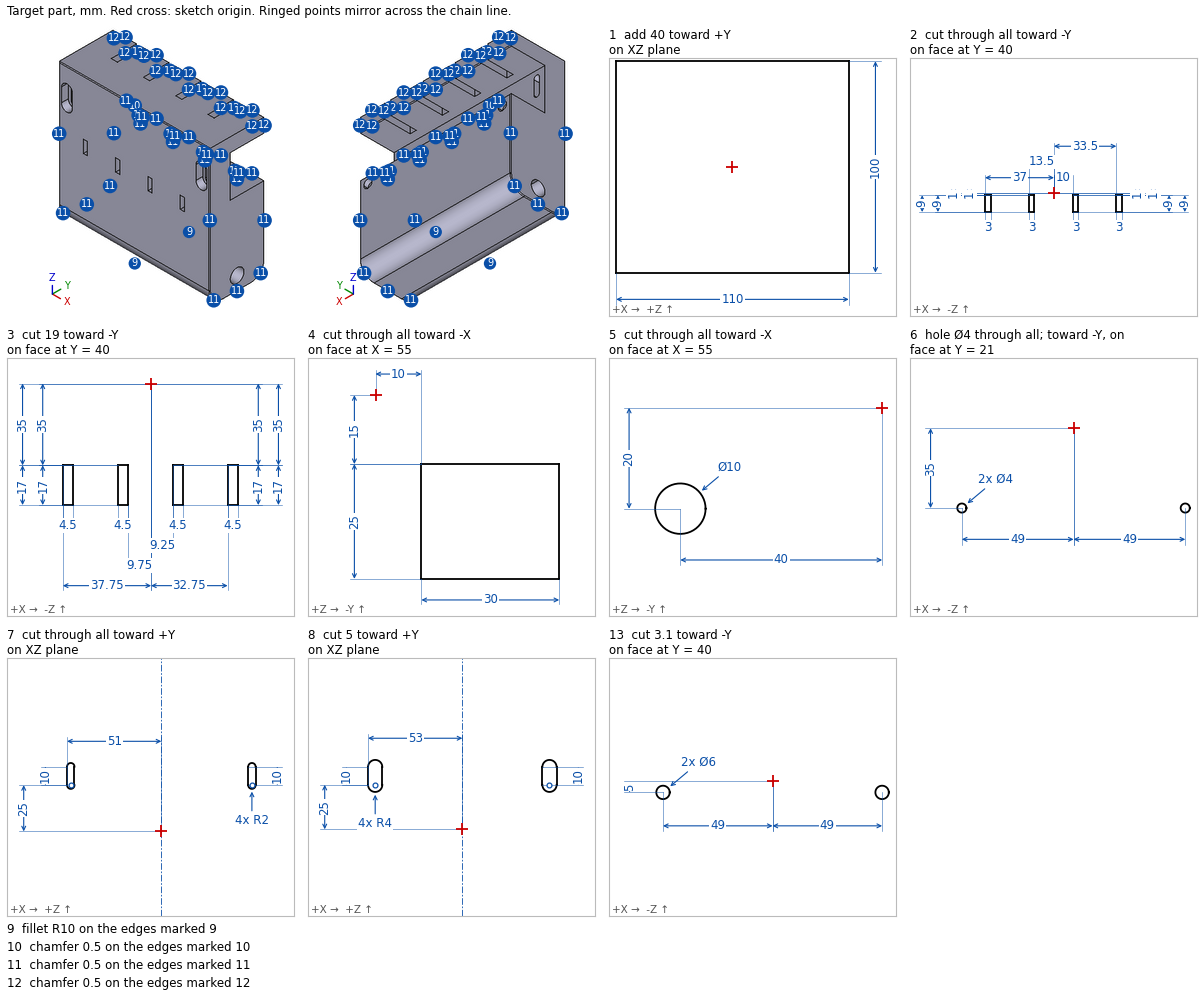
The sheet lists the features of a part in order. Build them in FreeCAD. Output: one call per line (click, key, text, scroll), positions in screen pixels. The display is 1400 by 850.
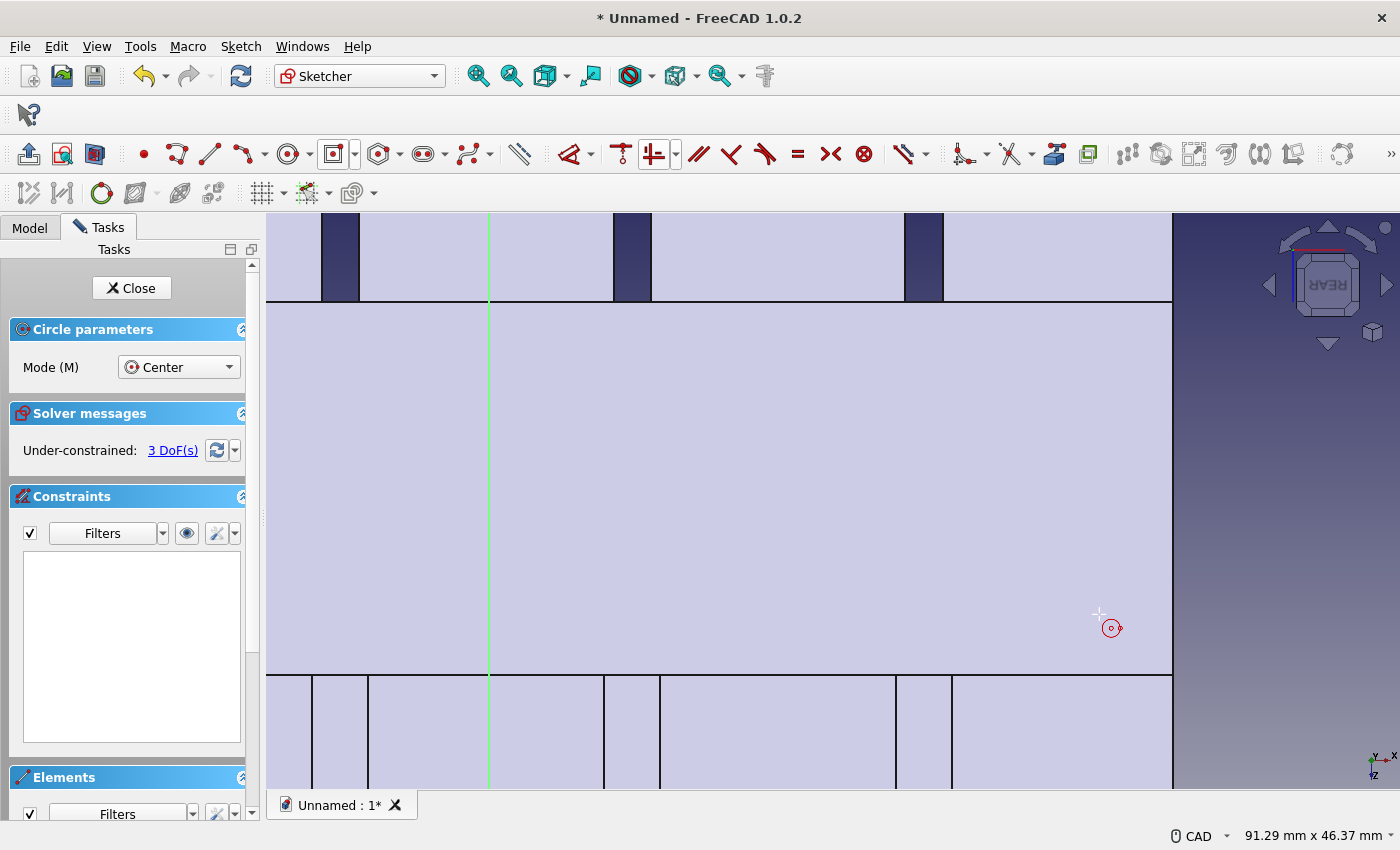
click(1098, 613)
click(1116, 595)
key(Escape)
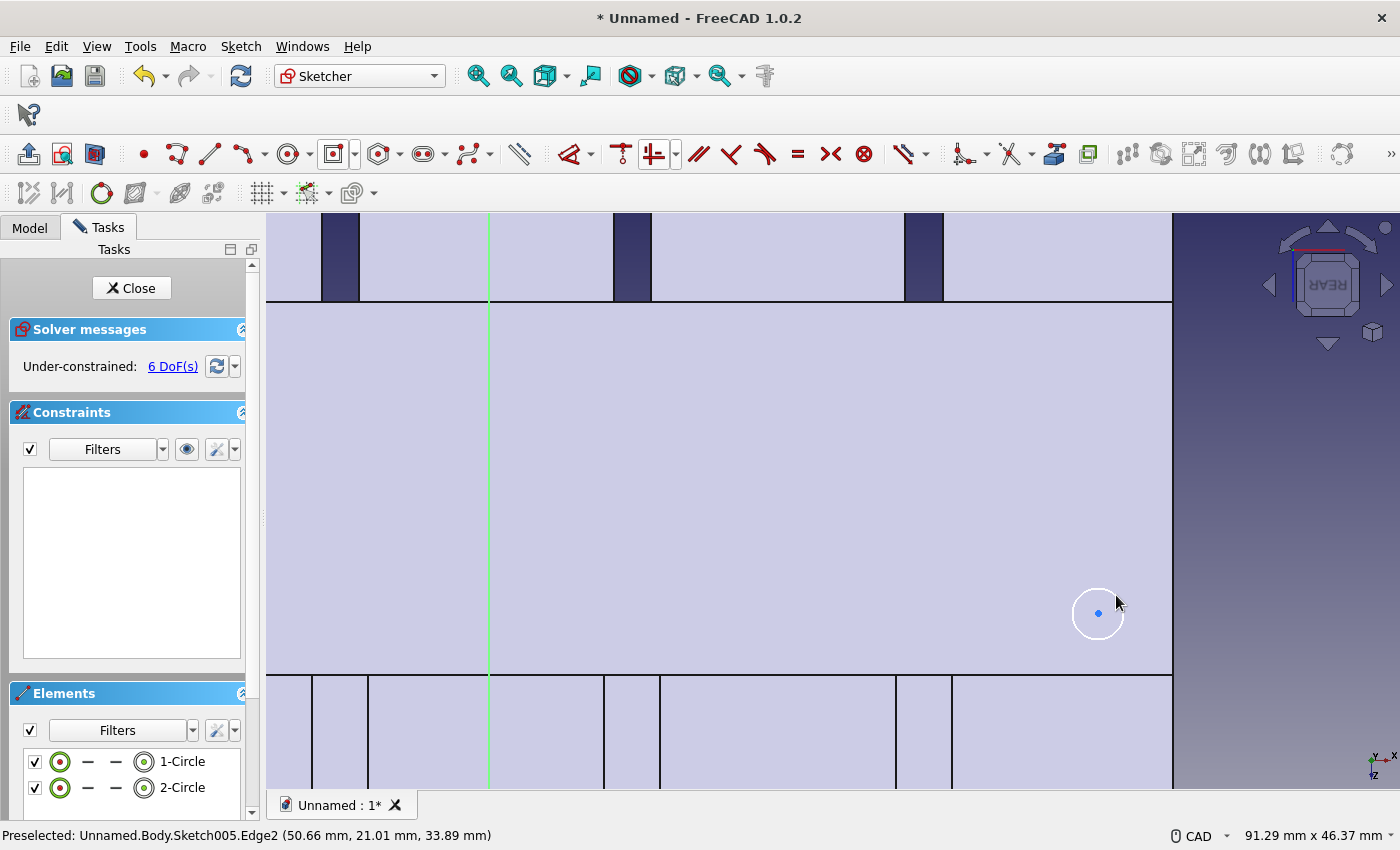
scroll(1099, 614, down, 3)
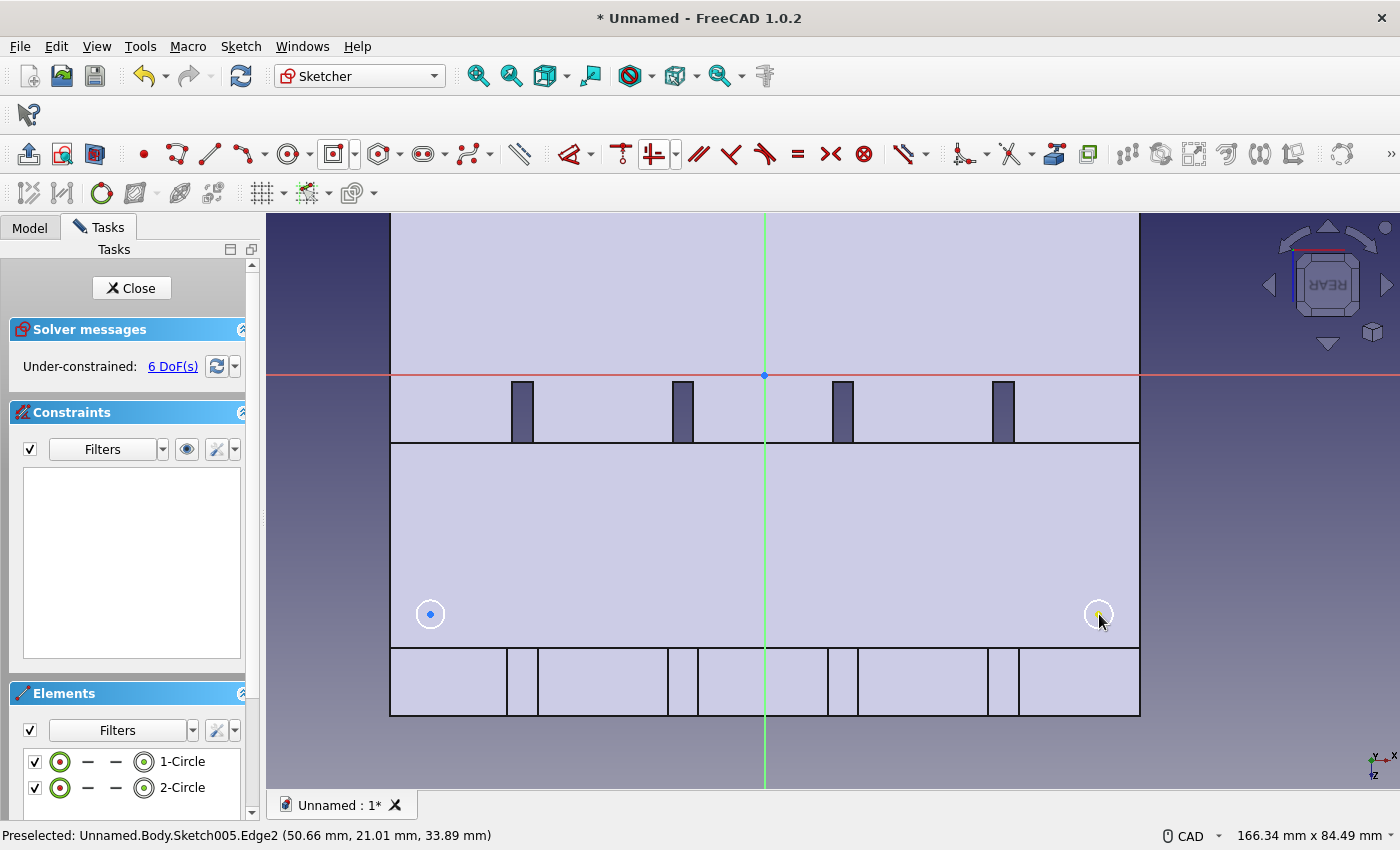
click(440, 604)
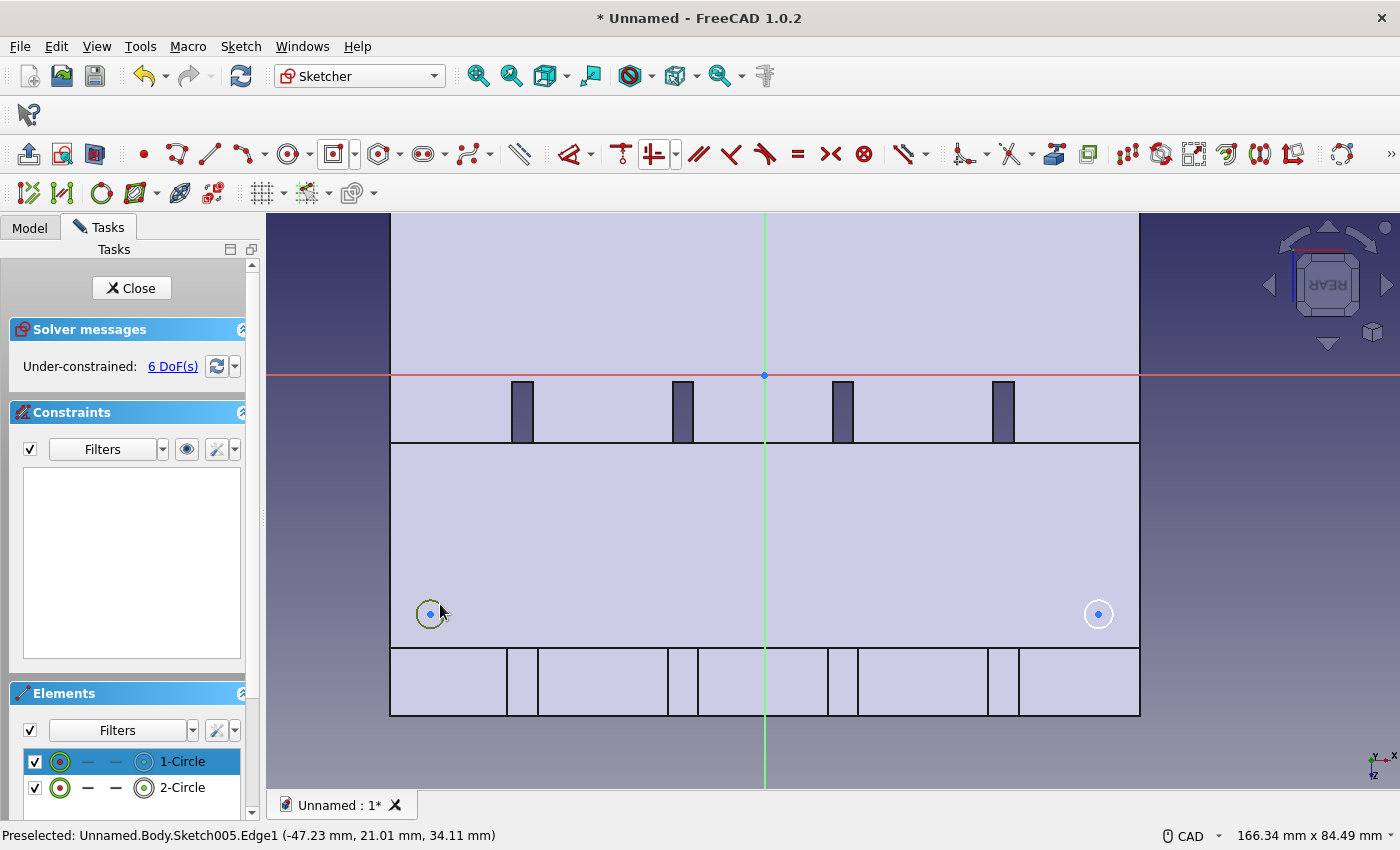
click(1109, 604)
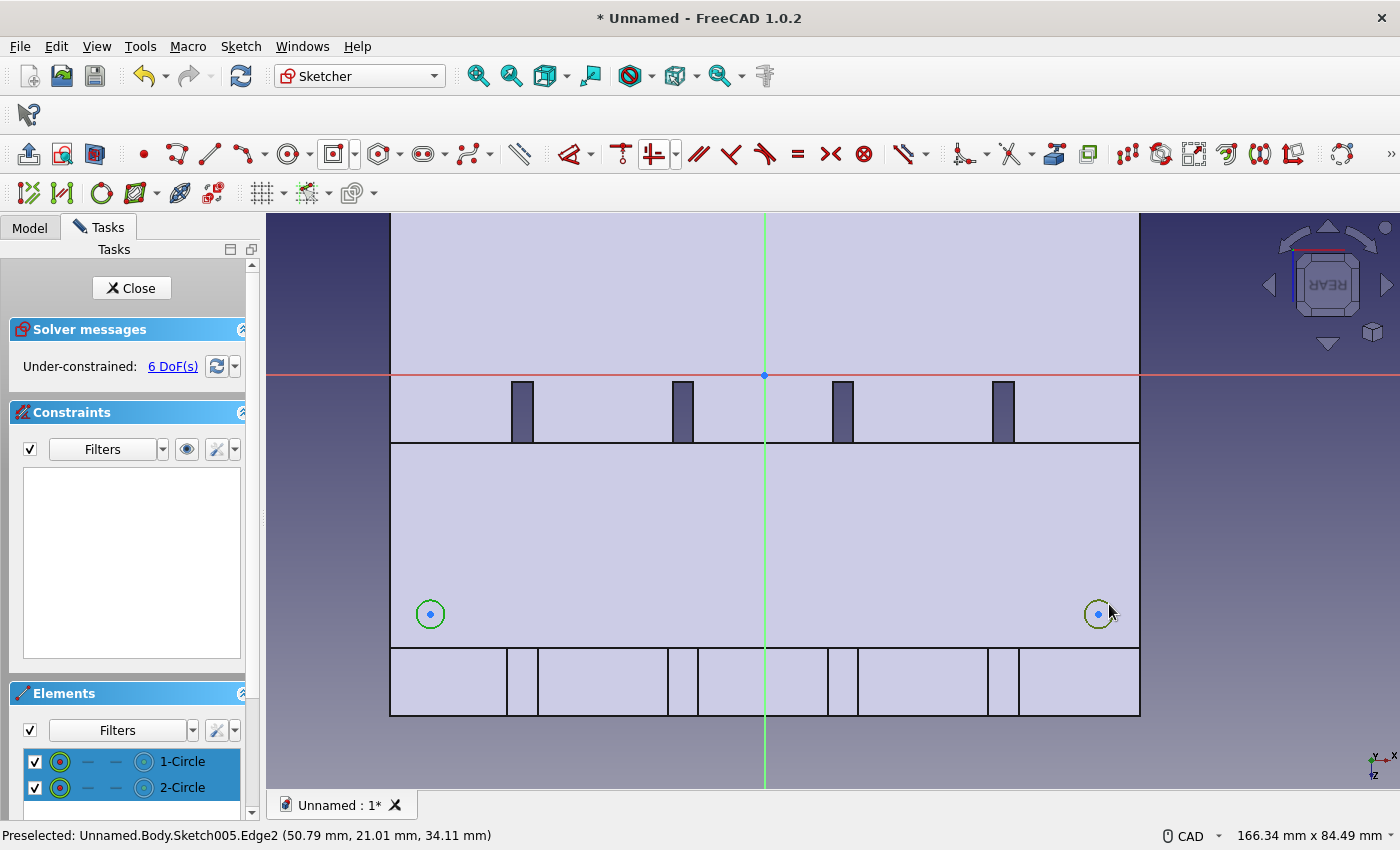
key(e)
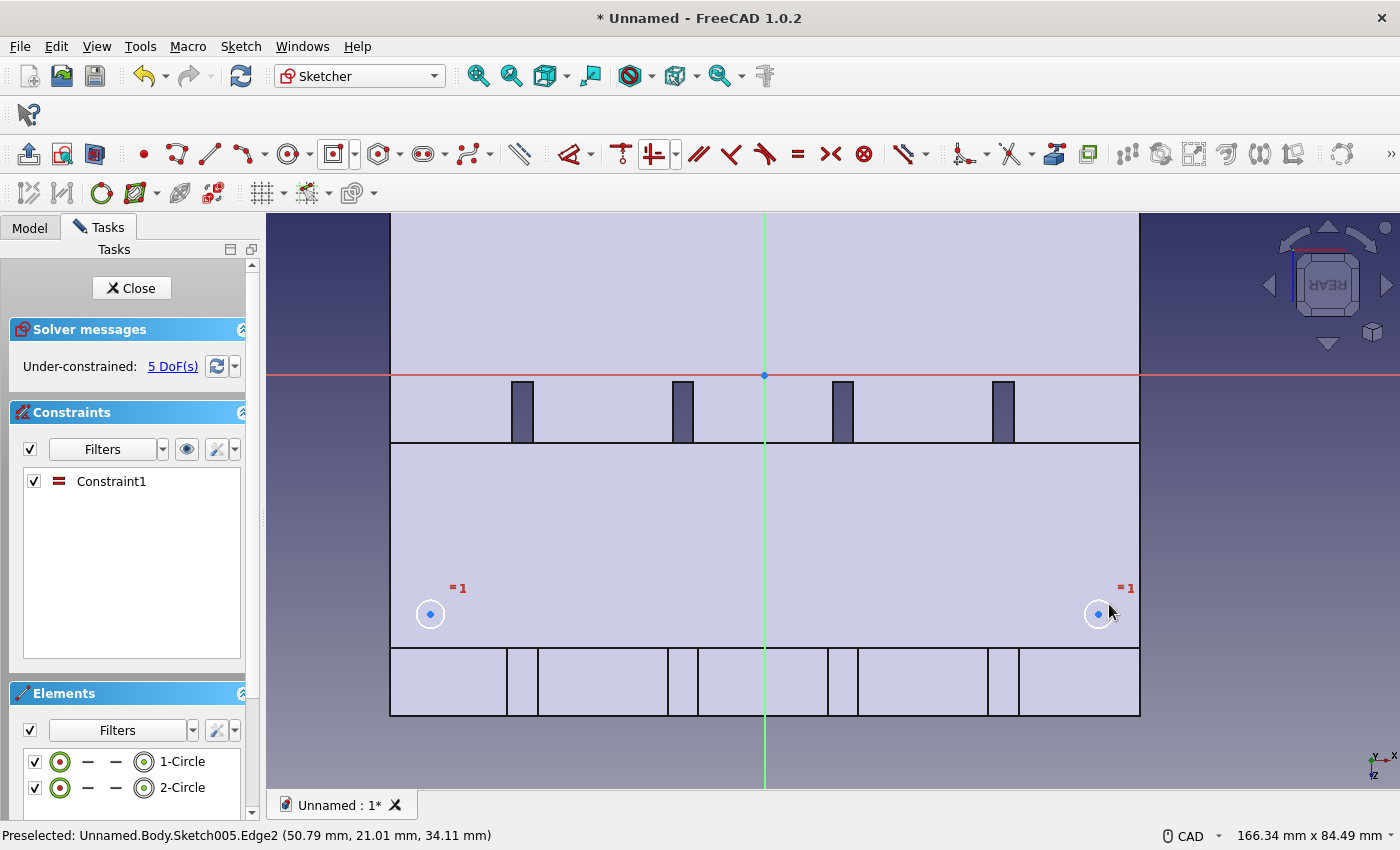
click(431, 614)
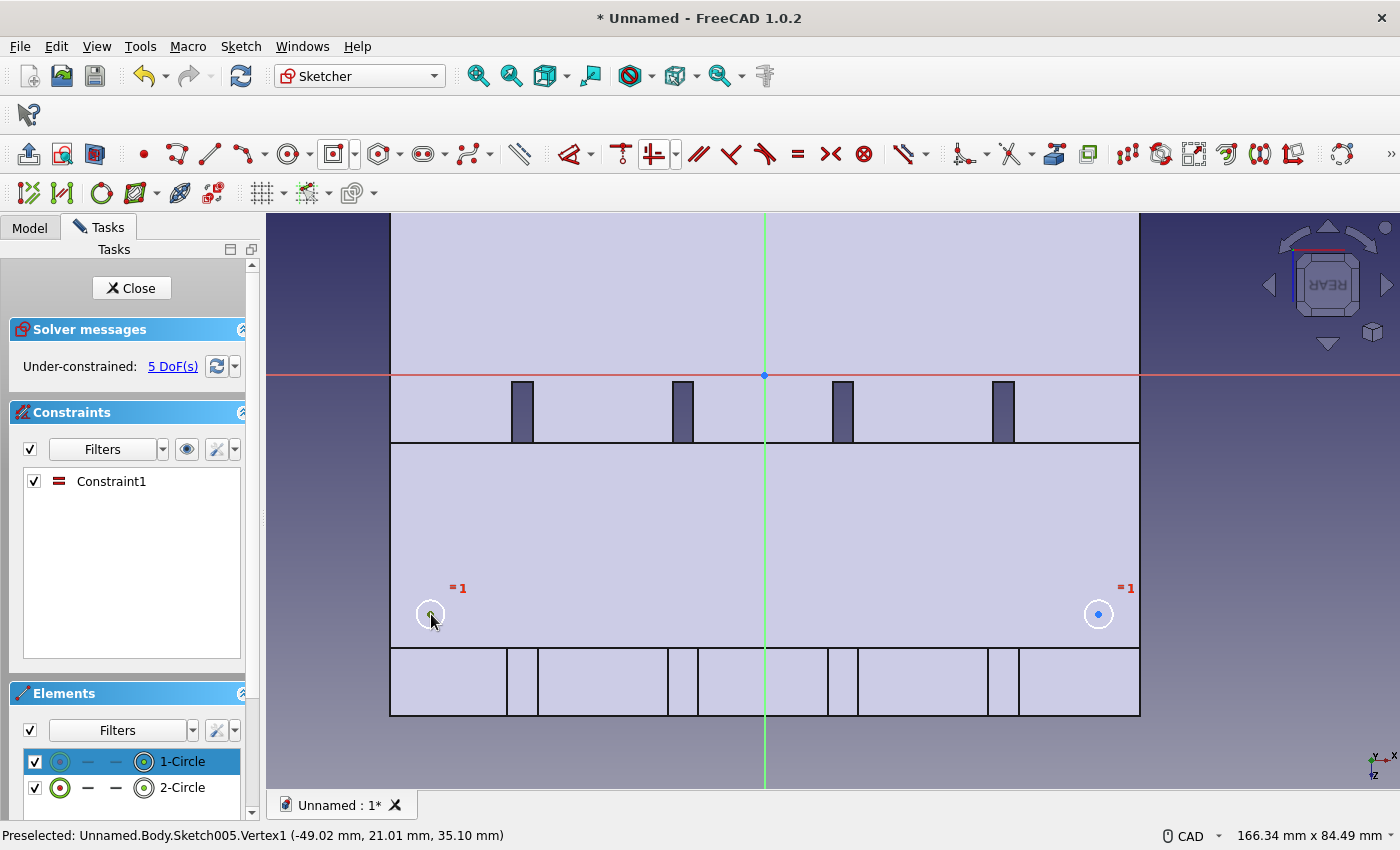
click(1099, 614)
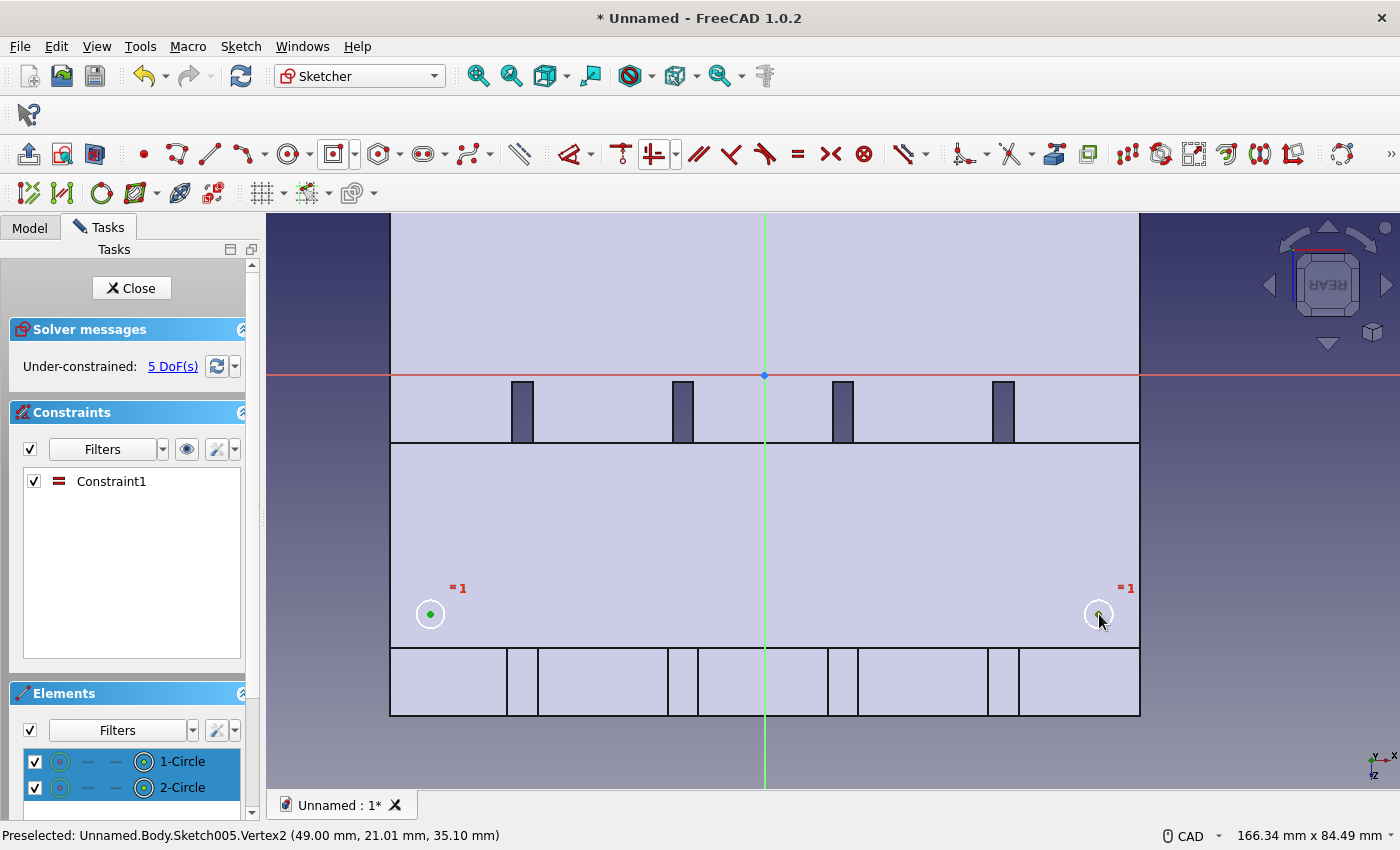
click(676, 154)